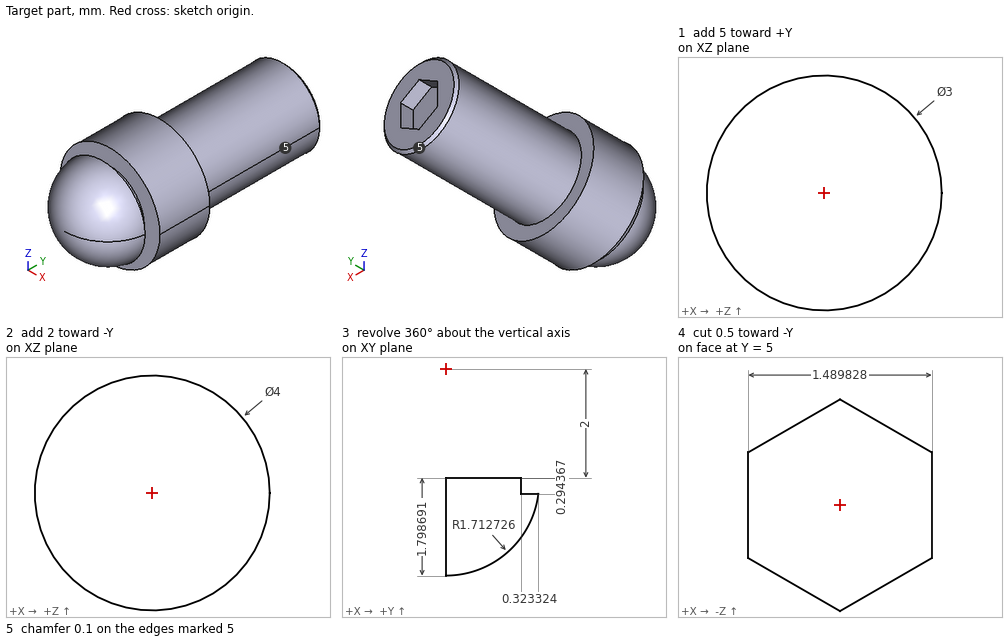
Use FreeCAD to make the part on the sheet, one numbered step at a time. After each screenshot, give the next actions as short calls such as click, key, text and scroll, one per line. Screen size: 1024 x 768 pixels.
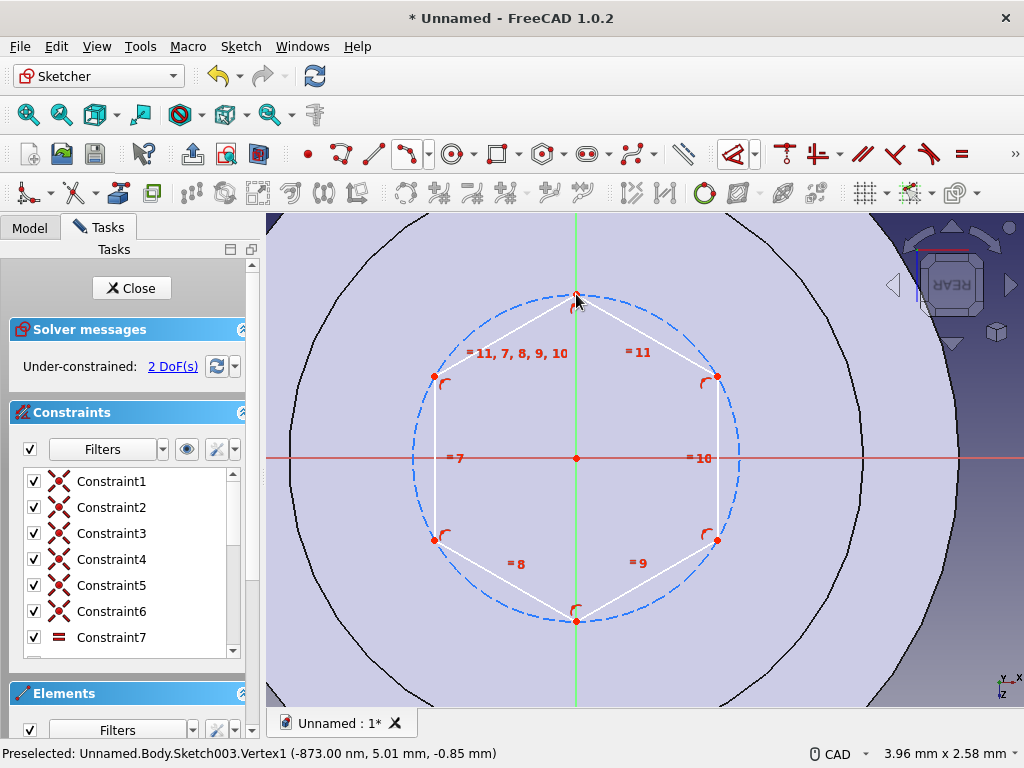
click(435, 426)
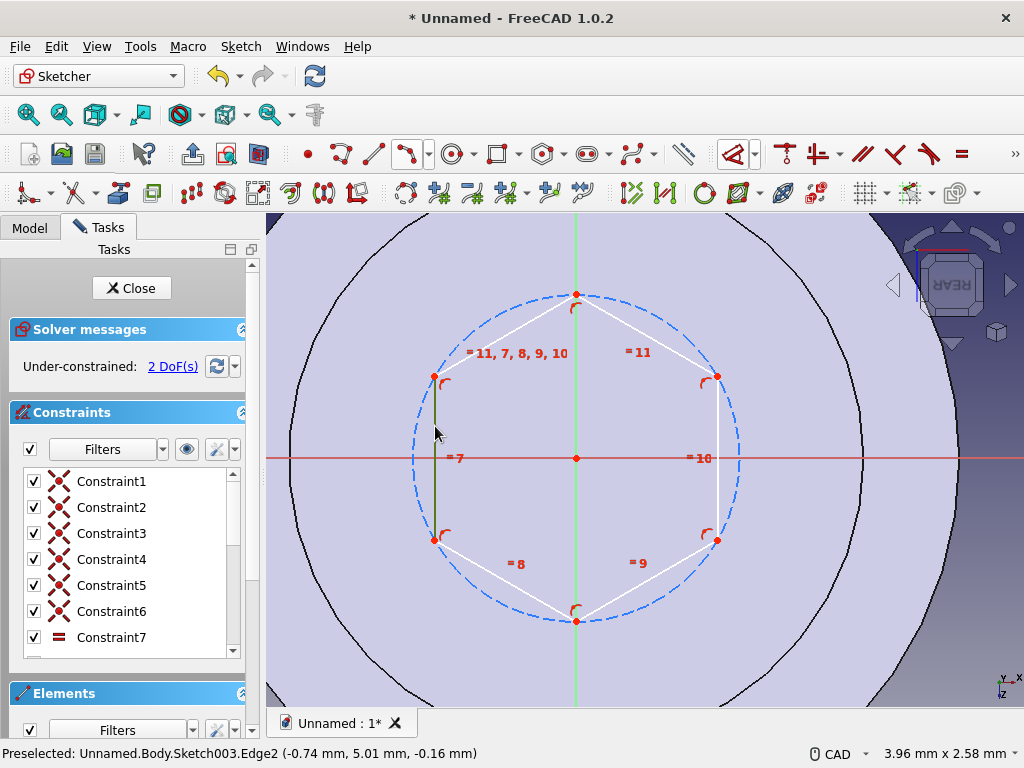
click(840, 154)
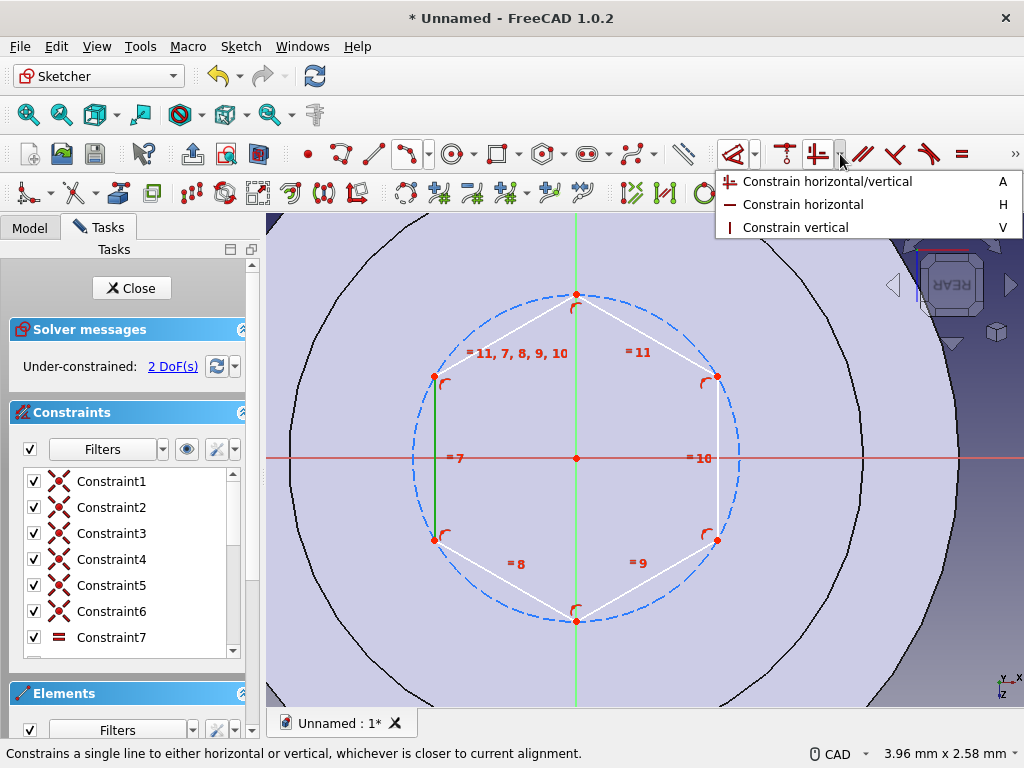
click(869, 228)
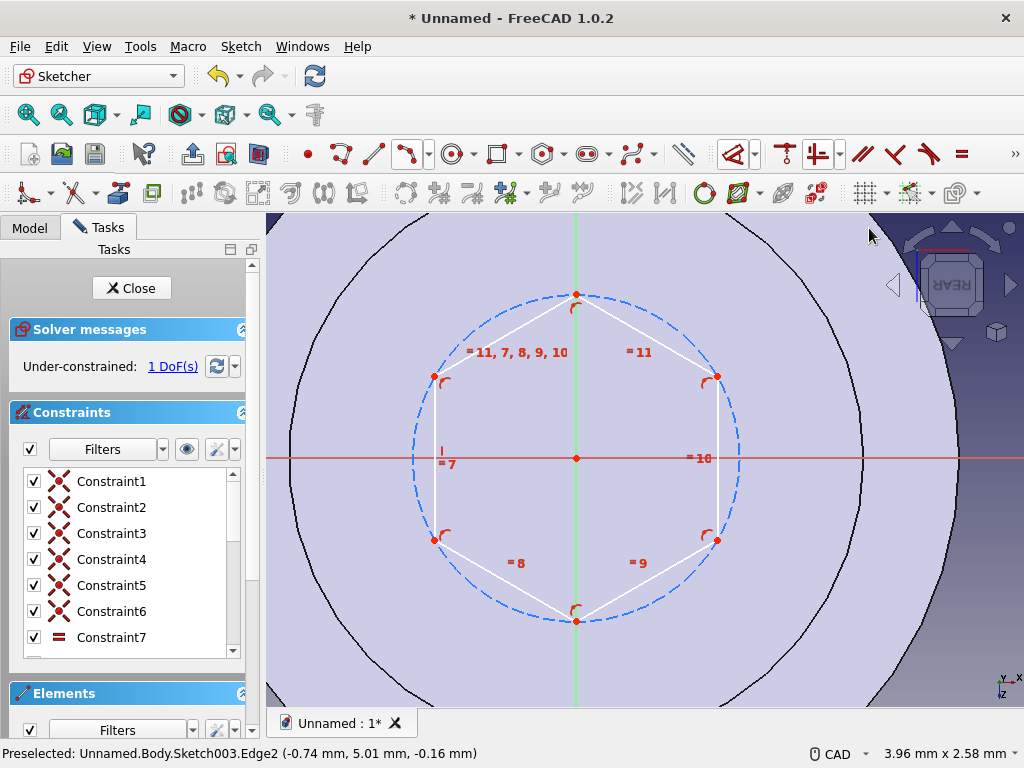
click(435, 377)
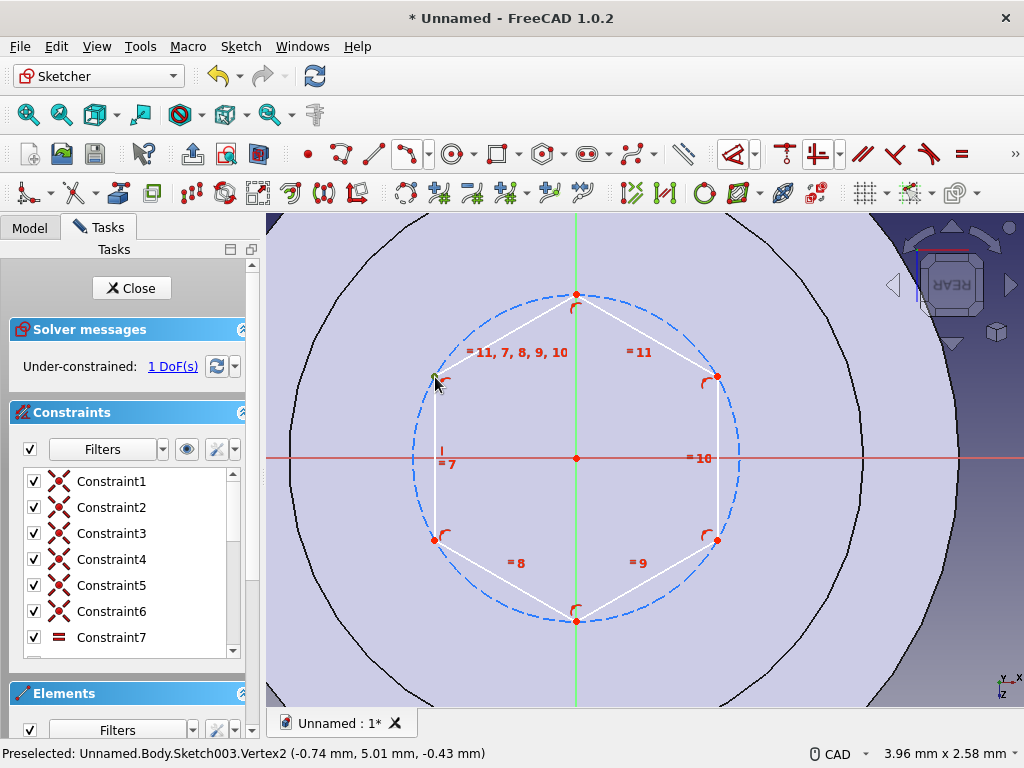
click(718, 540)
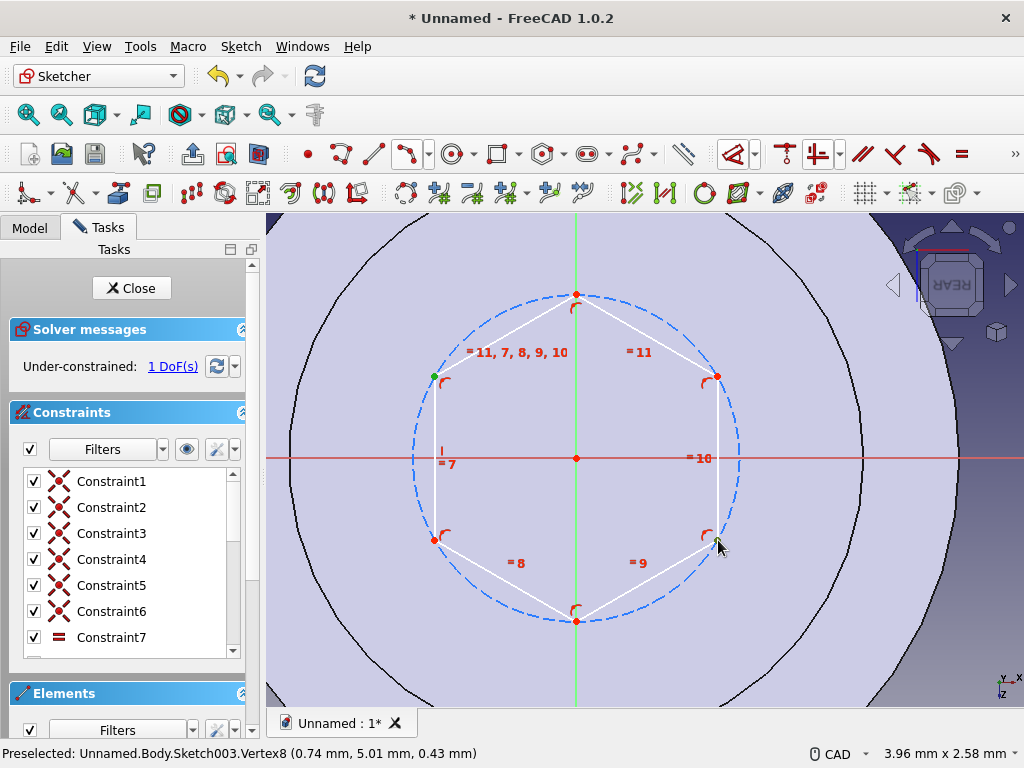
key(l)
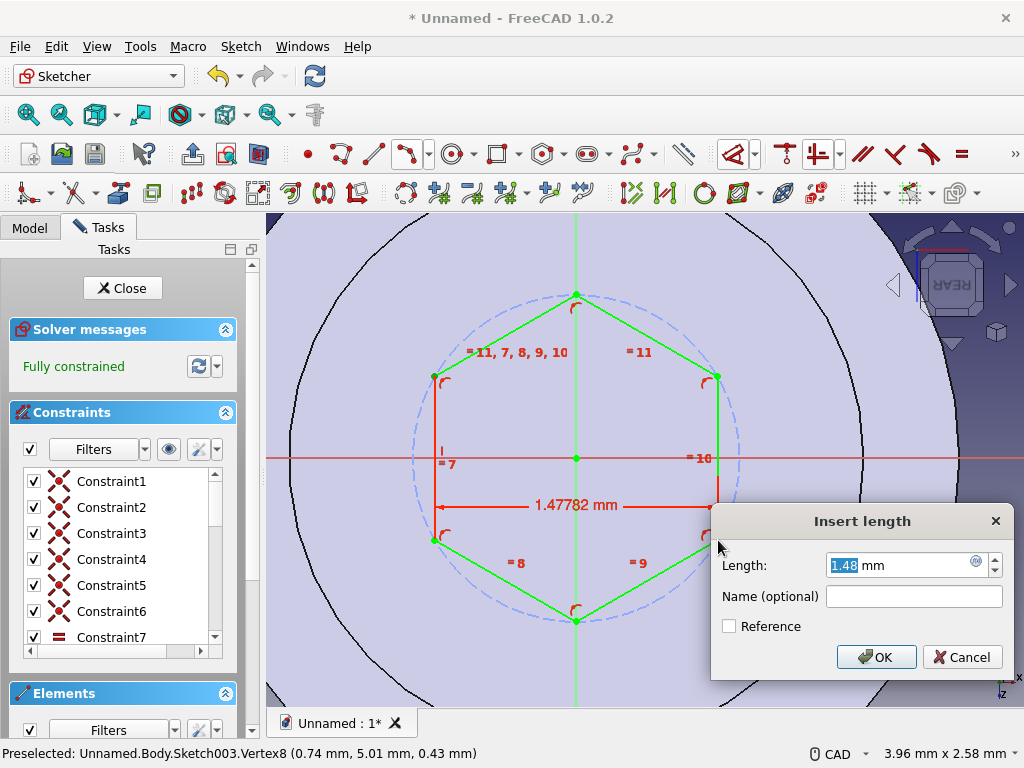
text(1.489828)
key(Return)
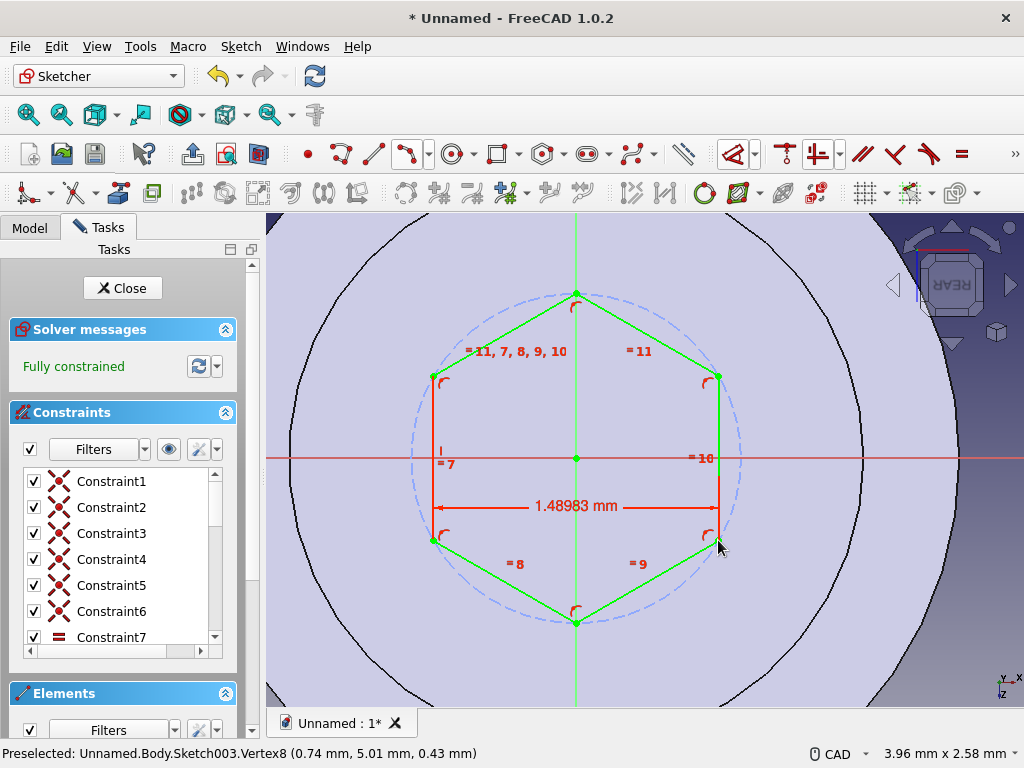
click(123, 288)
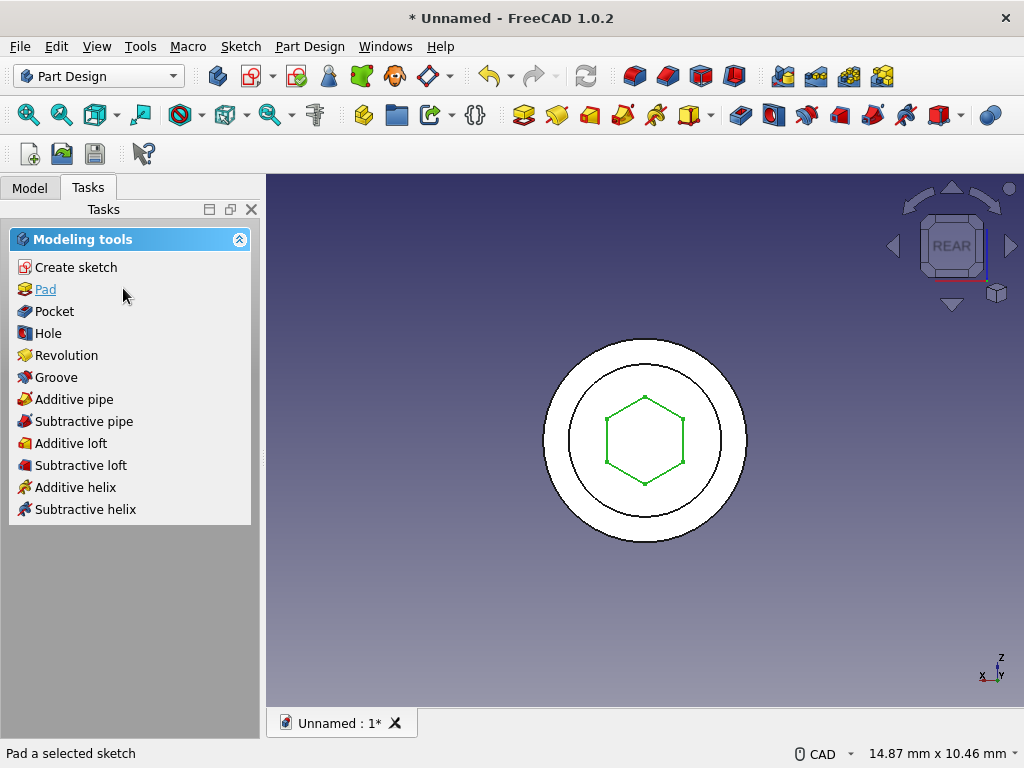
click(741, 116)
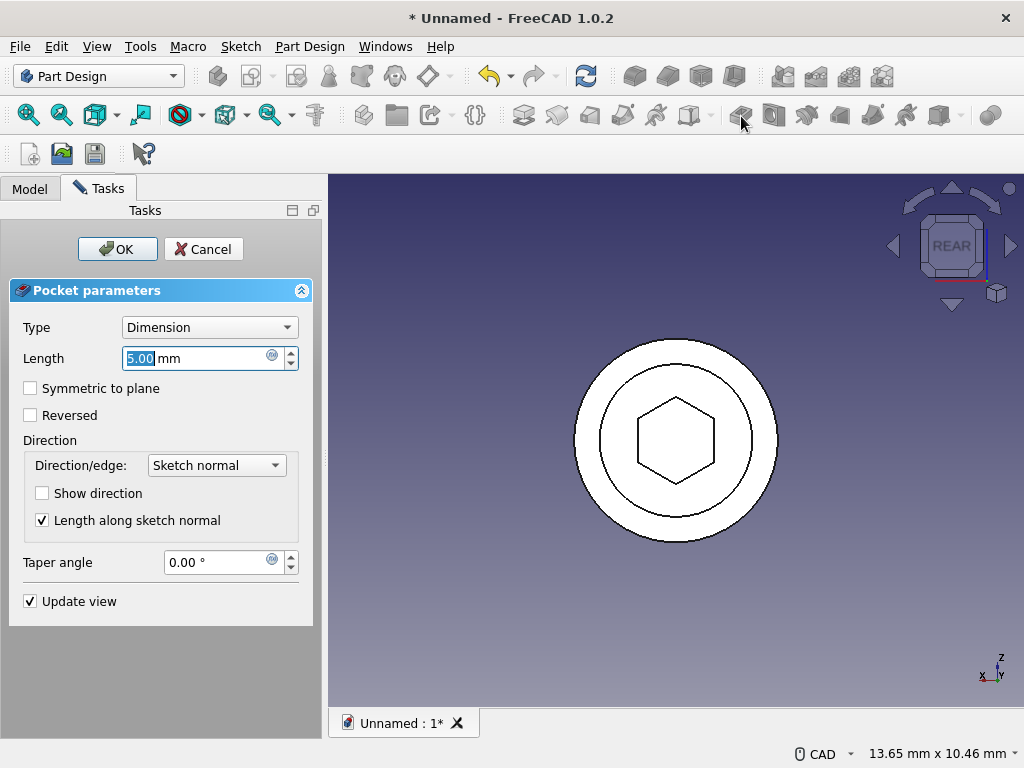
text(0.5)
key(Tab)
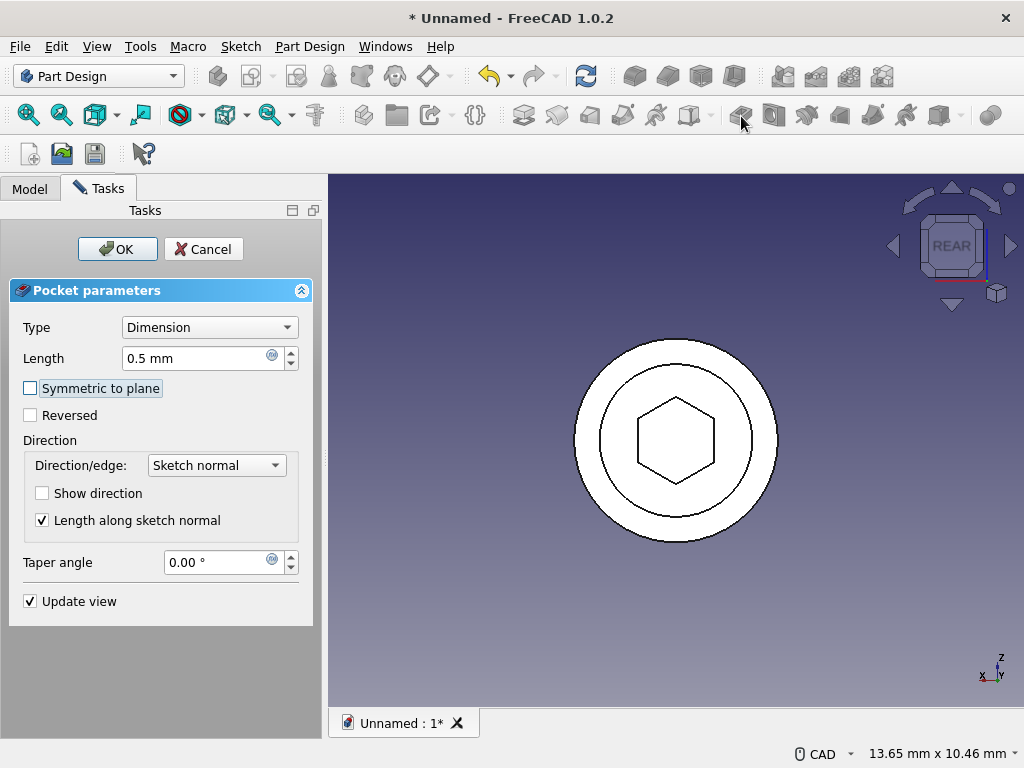
click(118, 249)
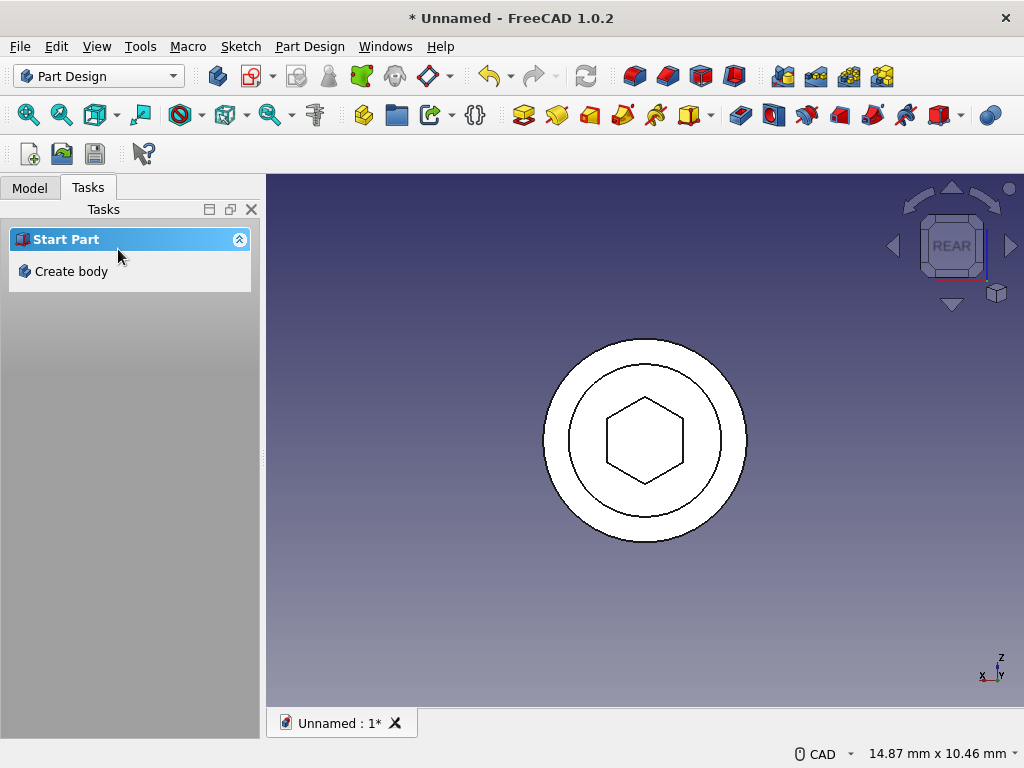
key(v)
key(f)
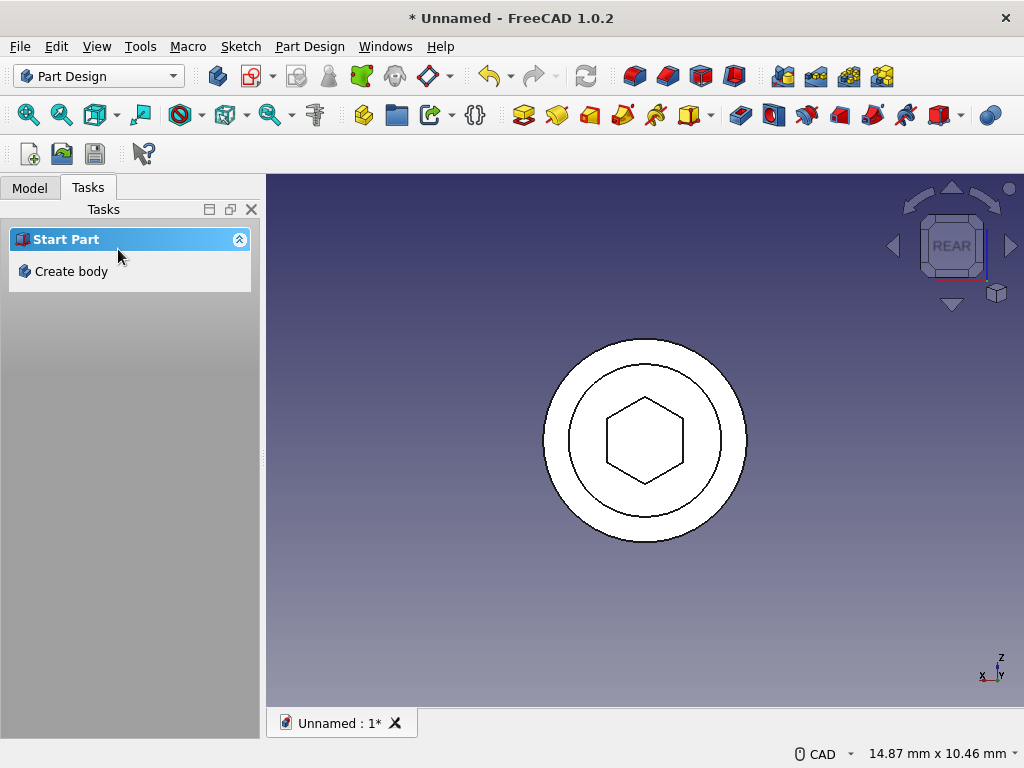
click(721, 439)